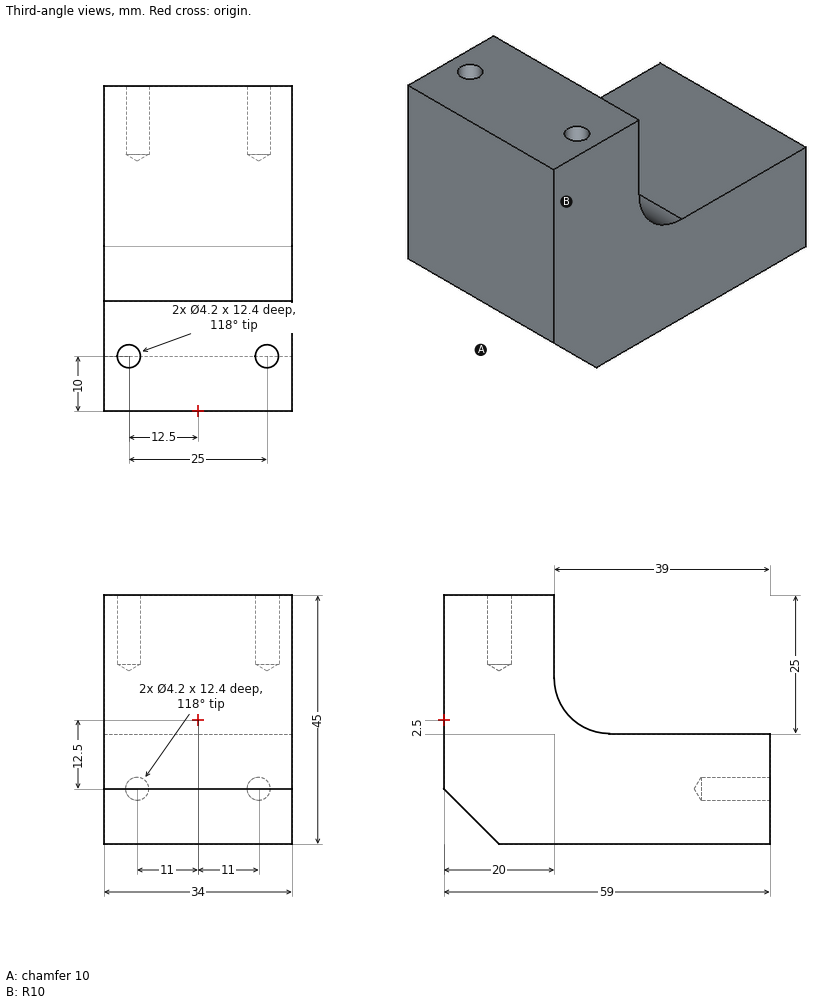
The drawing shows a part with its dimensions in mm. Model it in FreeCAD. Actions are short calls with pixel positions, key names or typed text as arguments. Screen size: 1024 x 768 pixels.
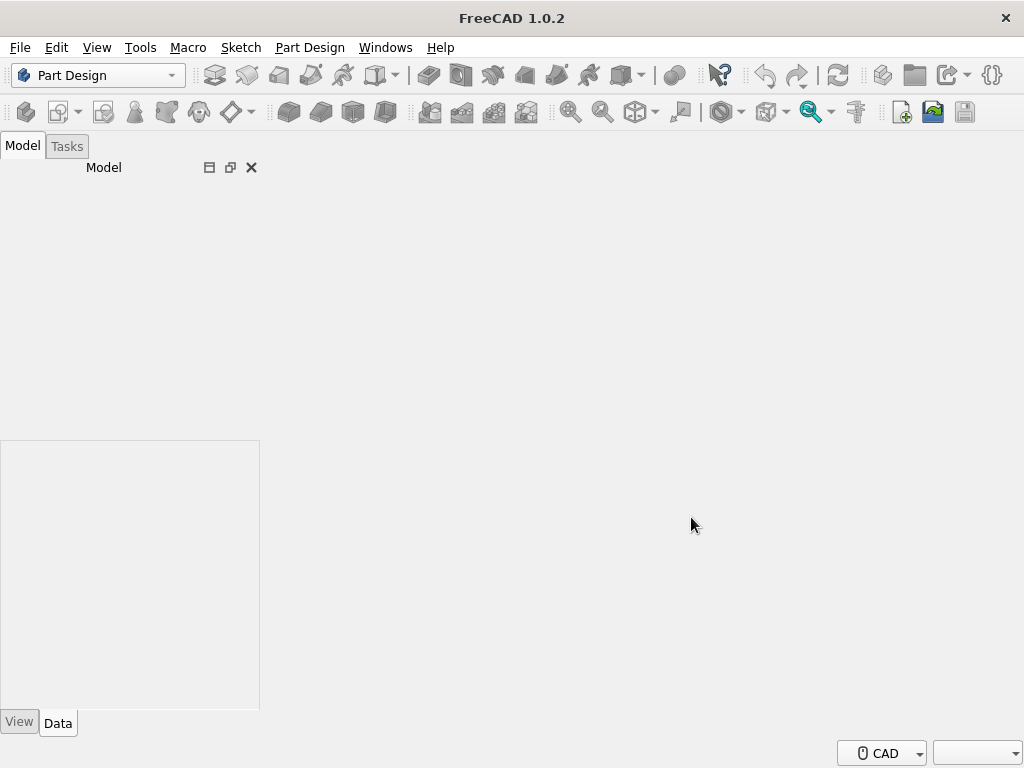
click(902, 112)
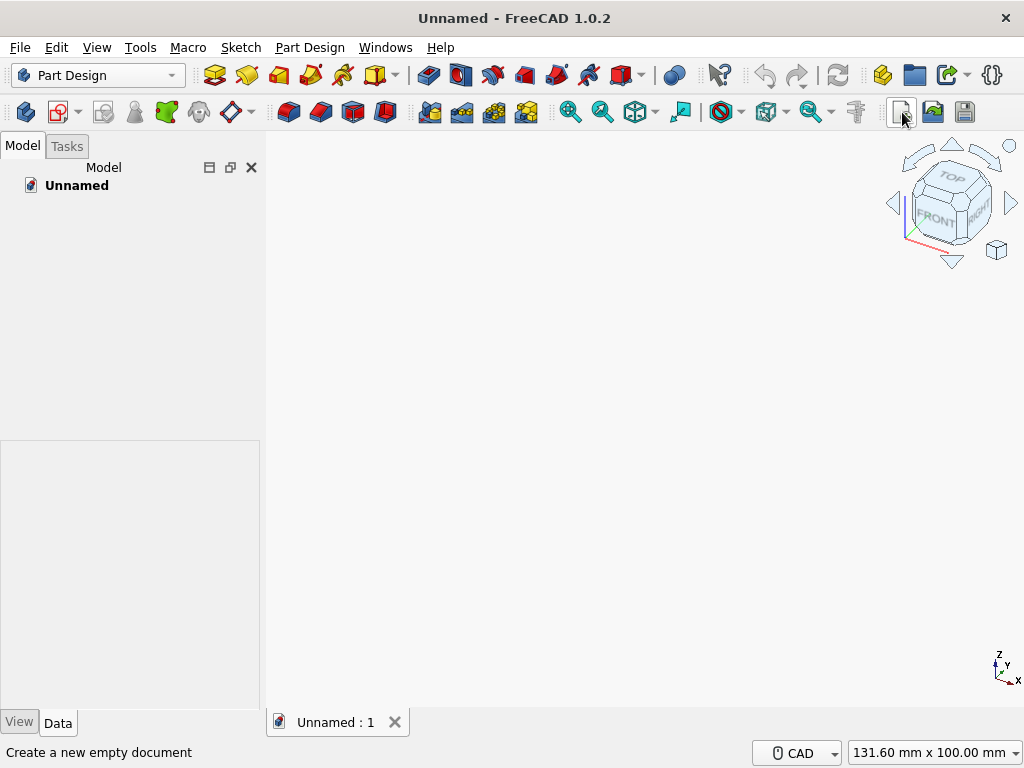
click(58, 112)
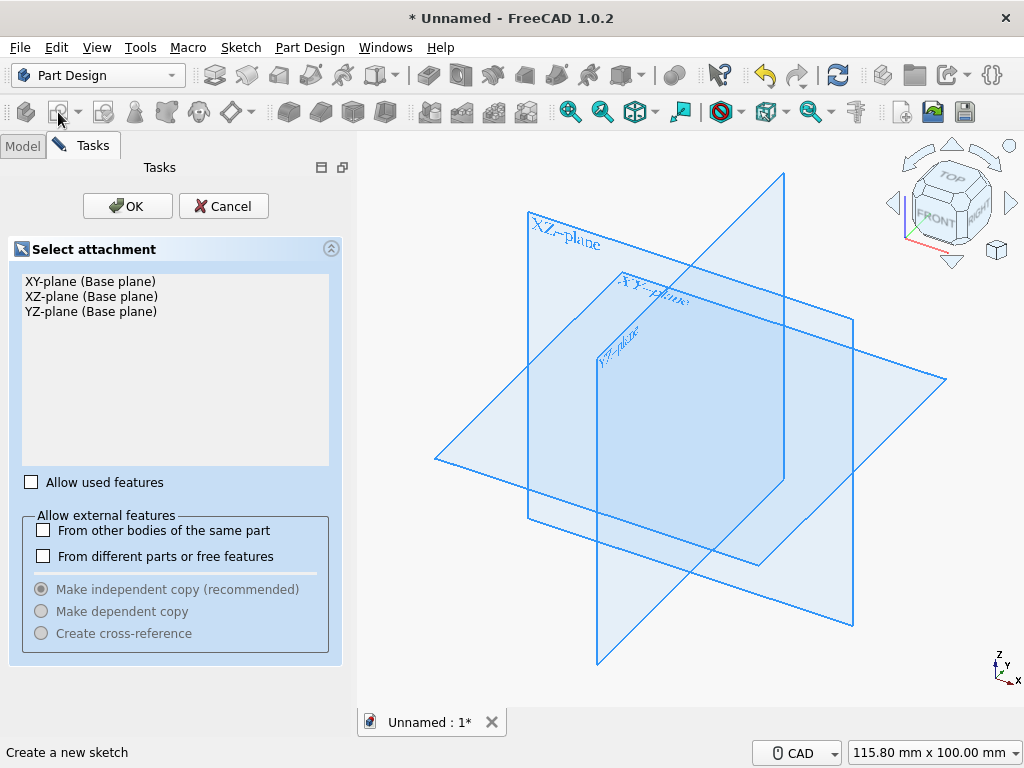
click(82, 296)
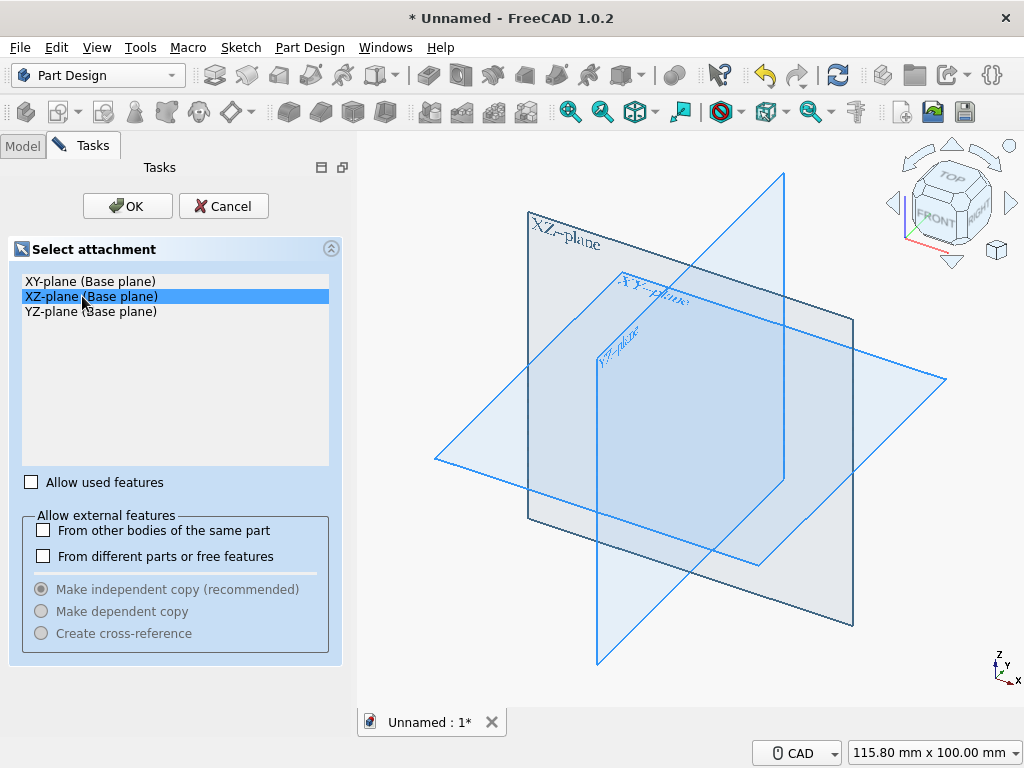
click(128, 206)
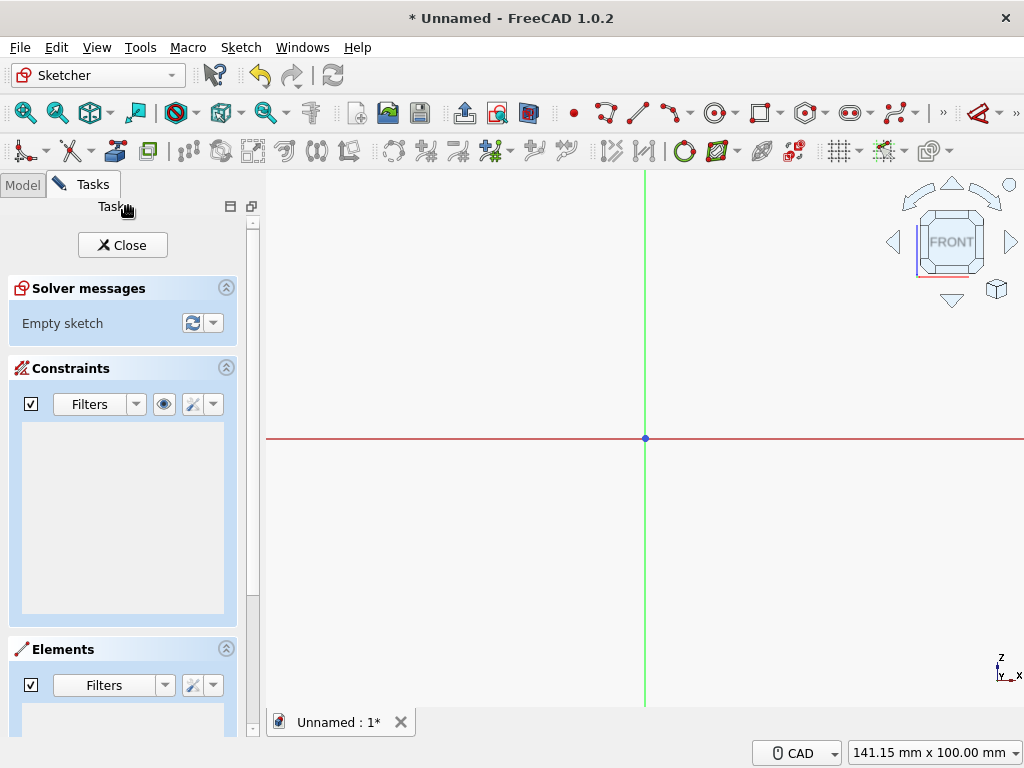
scroll(784, 439, up, 2)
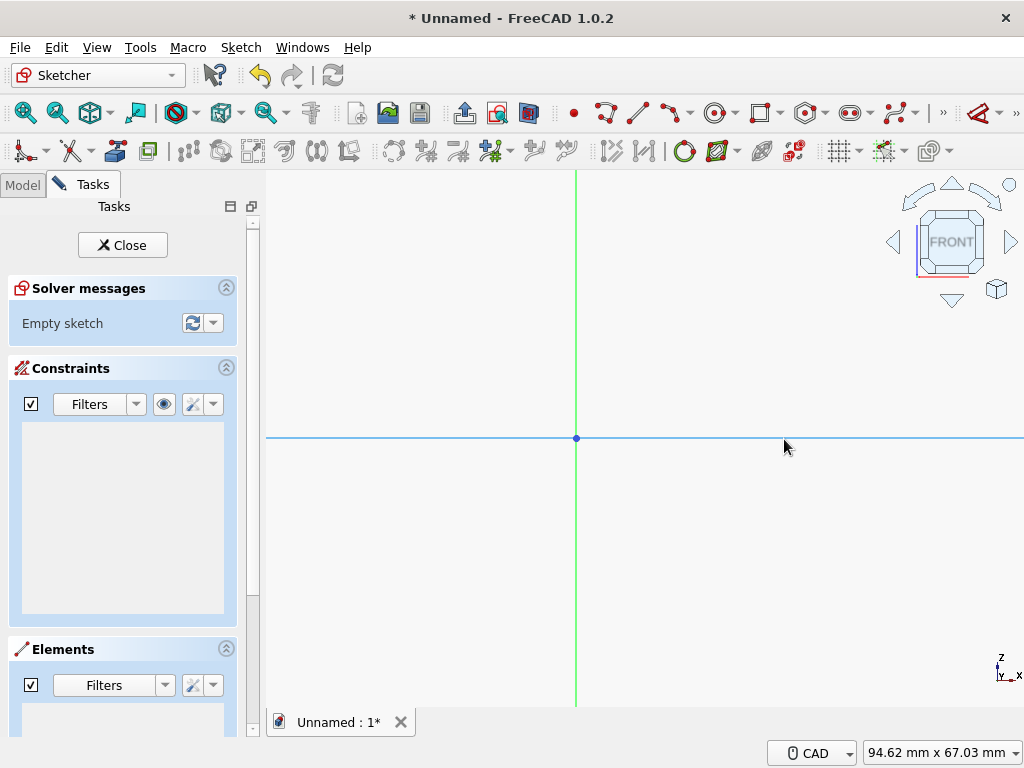
key(g)
key(v)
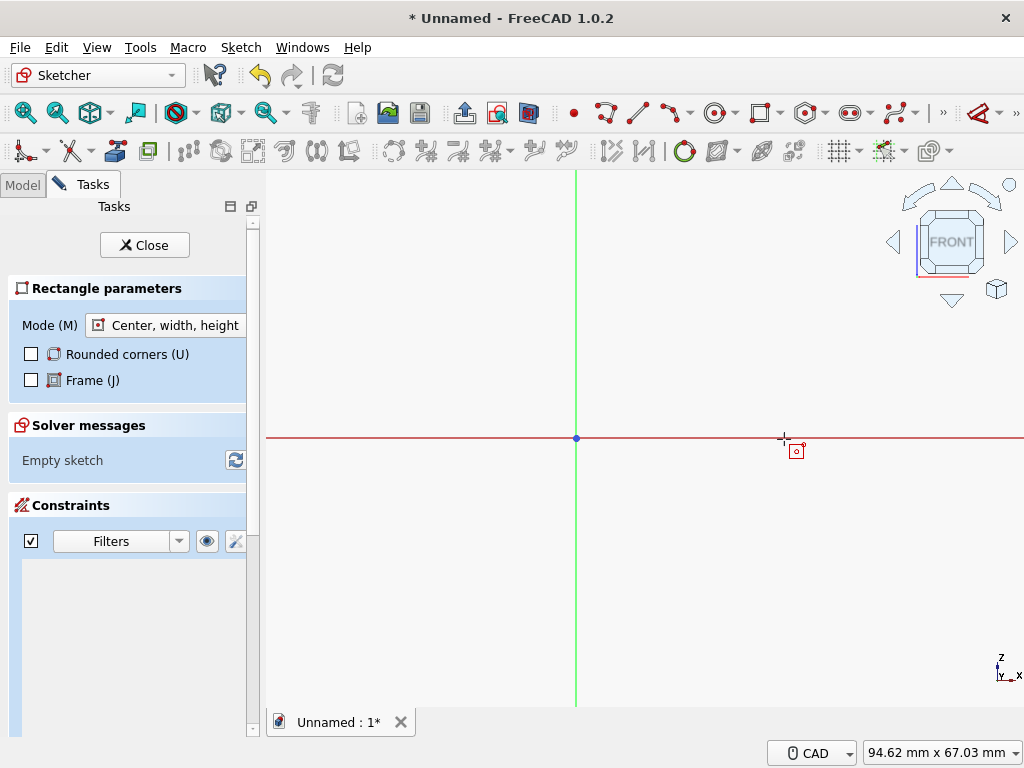
click(576, 438)
move(712, 258)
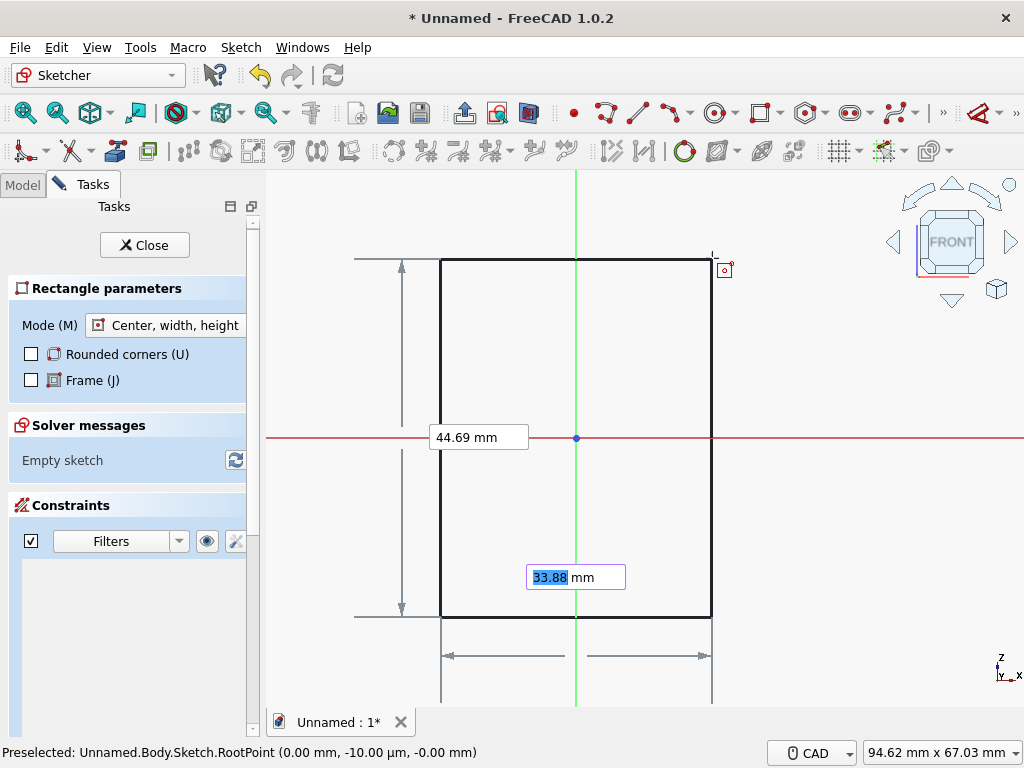
text(34)
key(Tab)
text(45)
key(Return)
key(Escape)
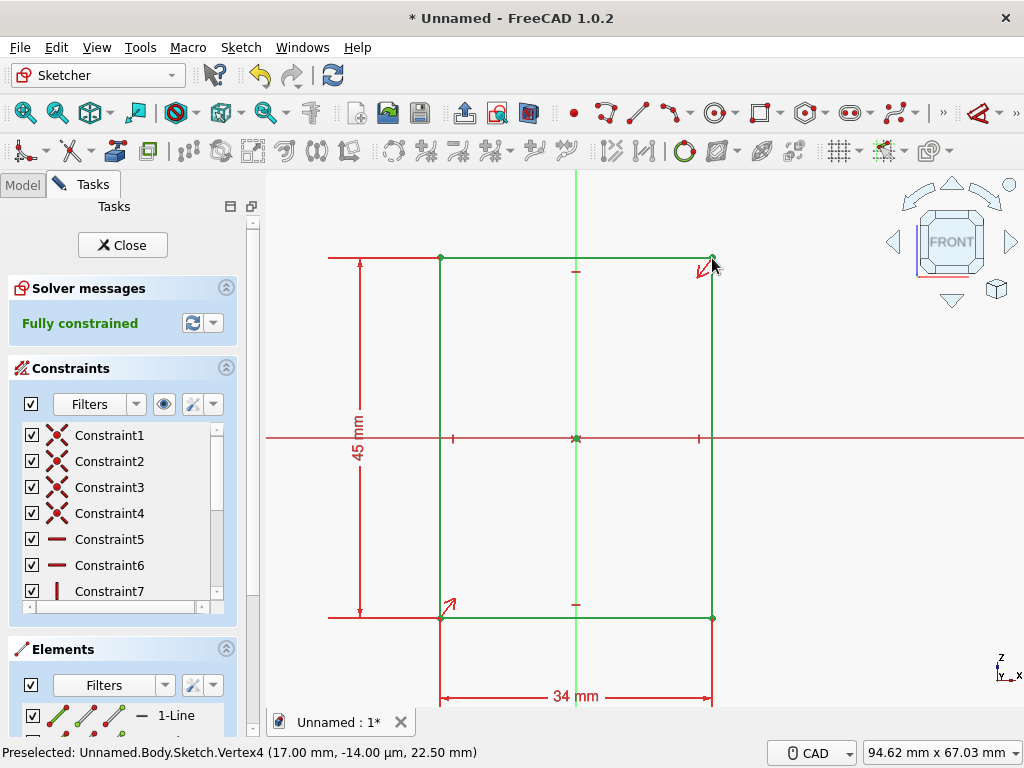
click(123, 245)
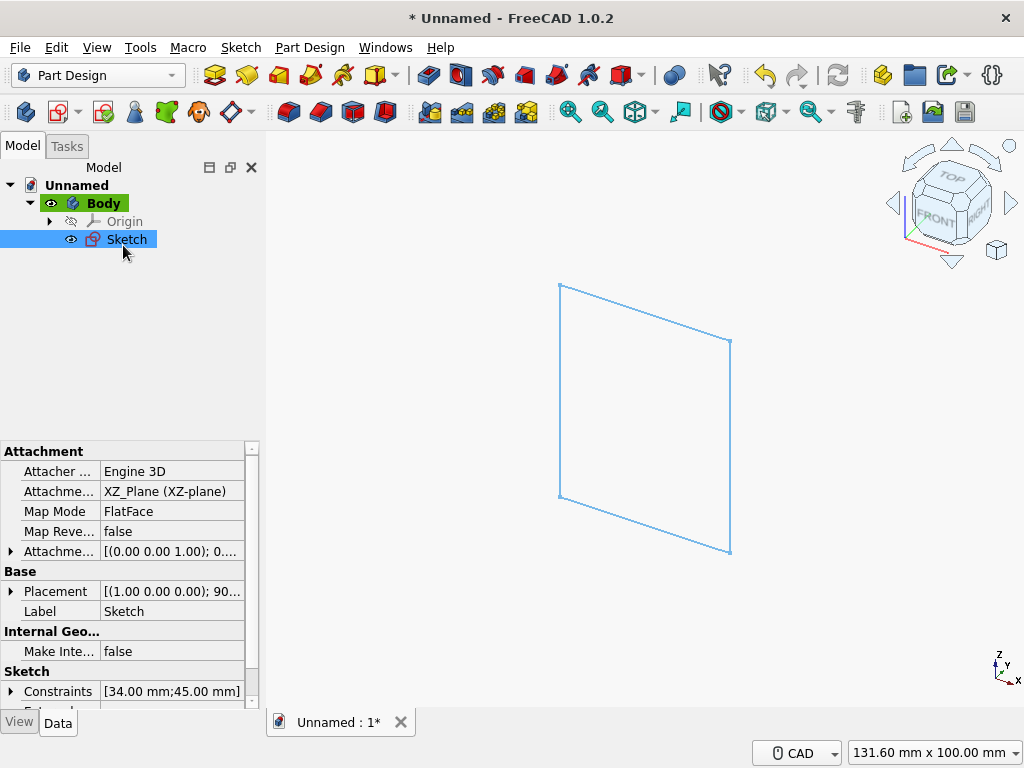
click(216, 76)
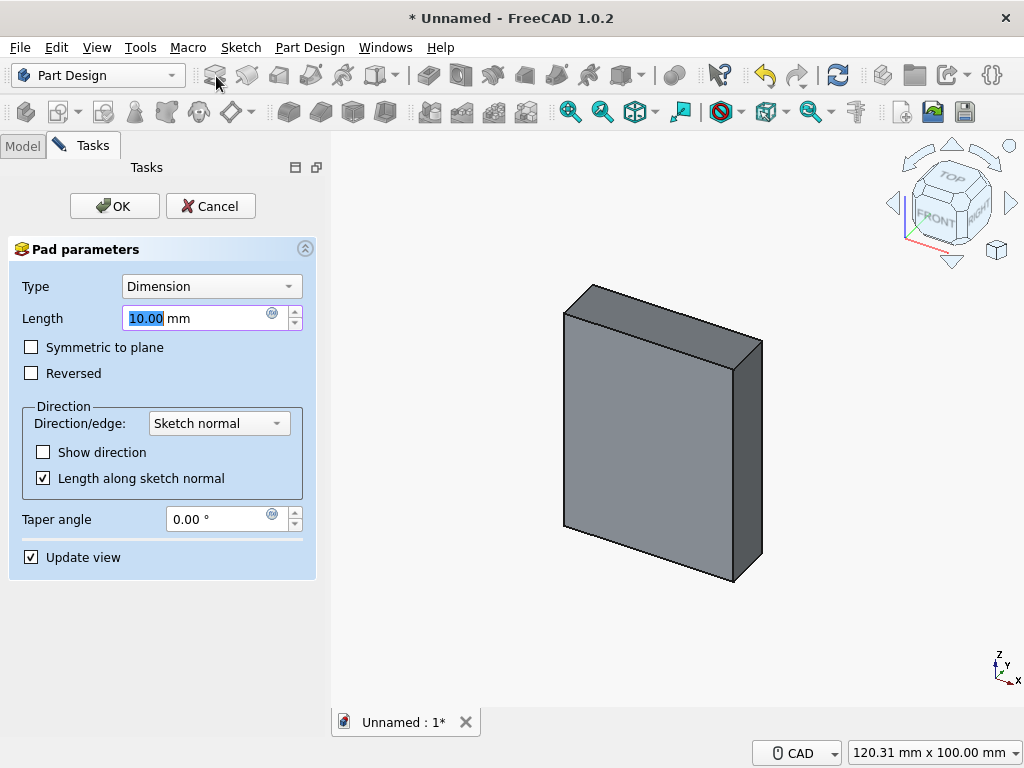
text(59)
key(Tab)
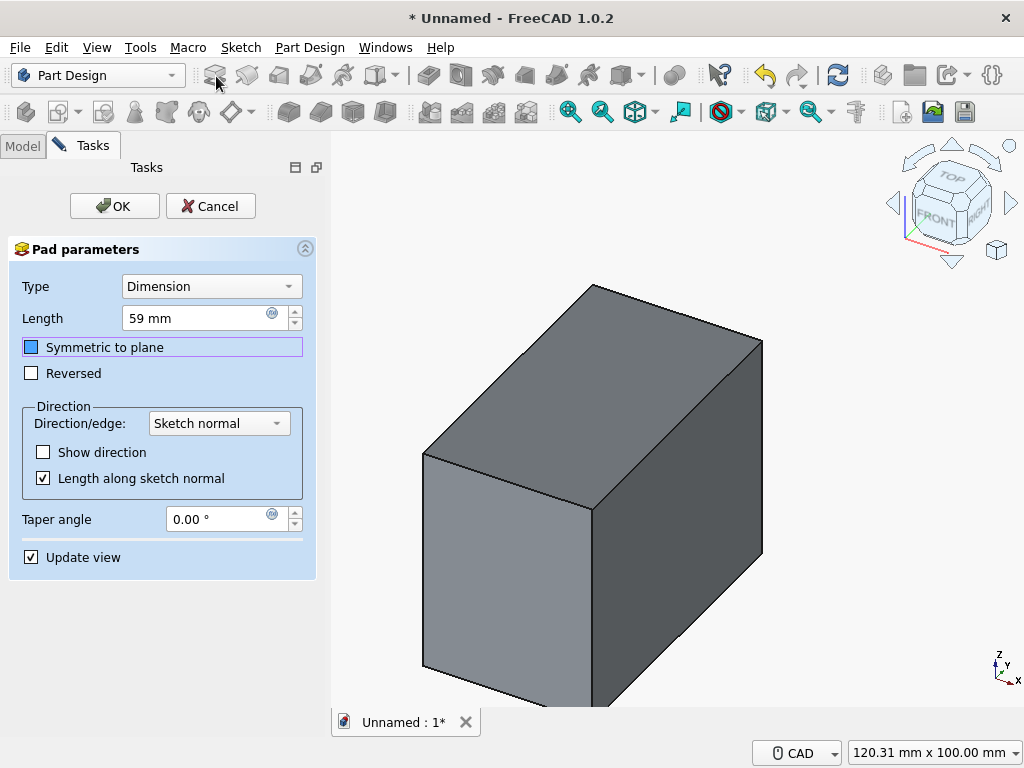
click(30, 373)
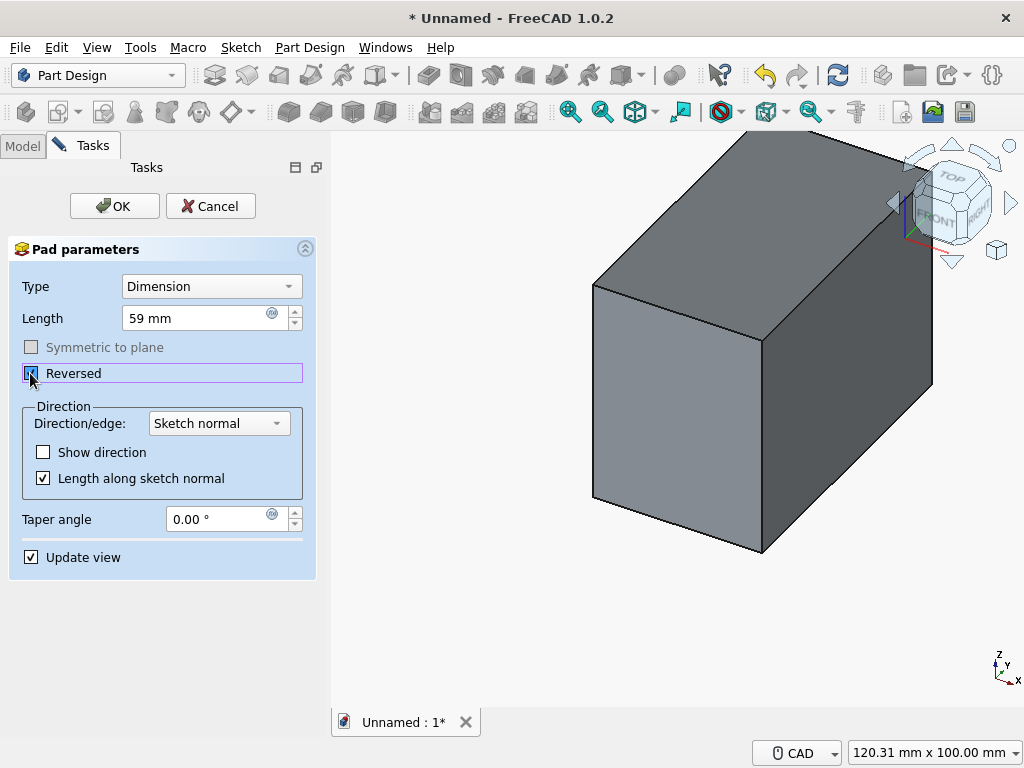
click(115, 206)